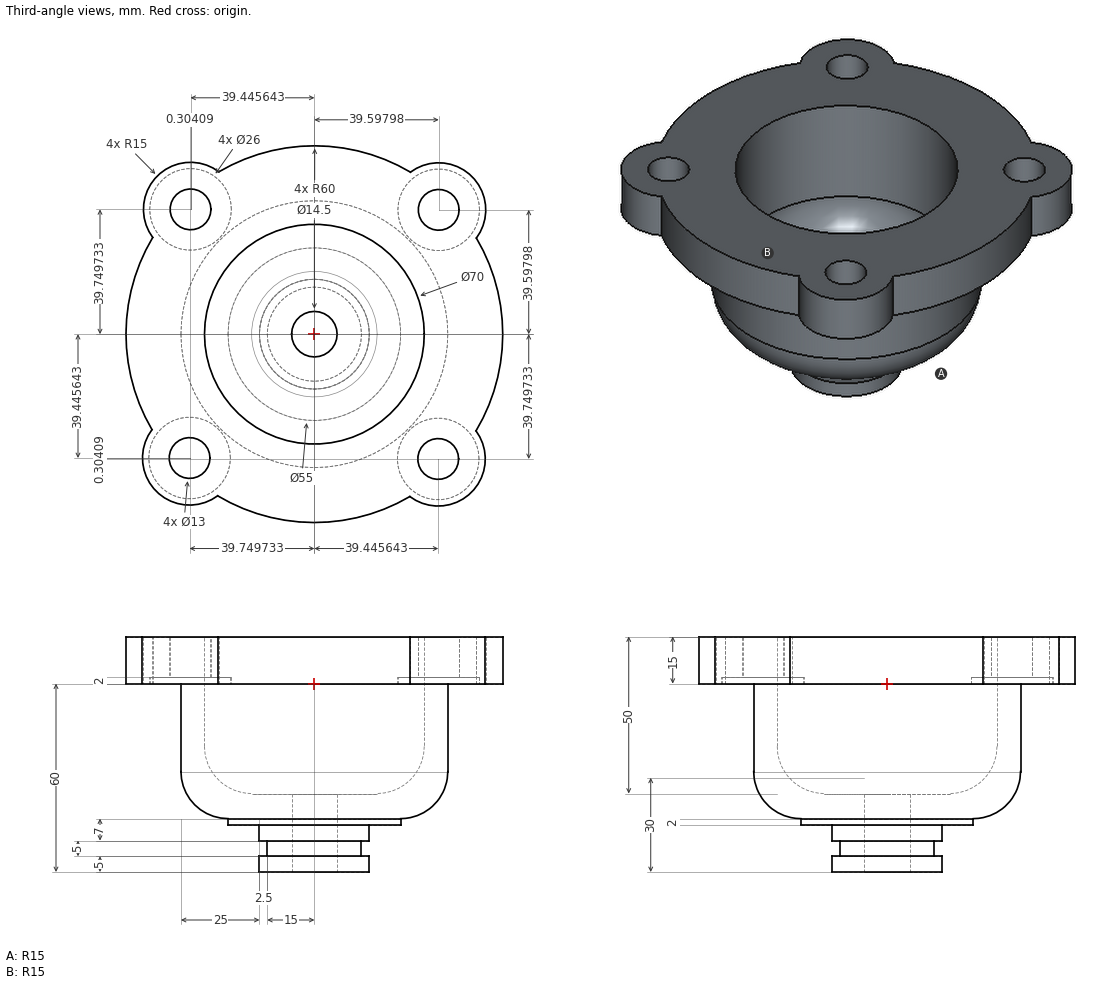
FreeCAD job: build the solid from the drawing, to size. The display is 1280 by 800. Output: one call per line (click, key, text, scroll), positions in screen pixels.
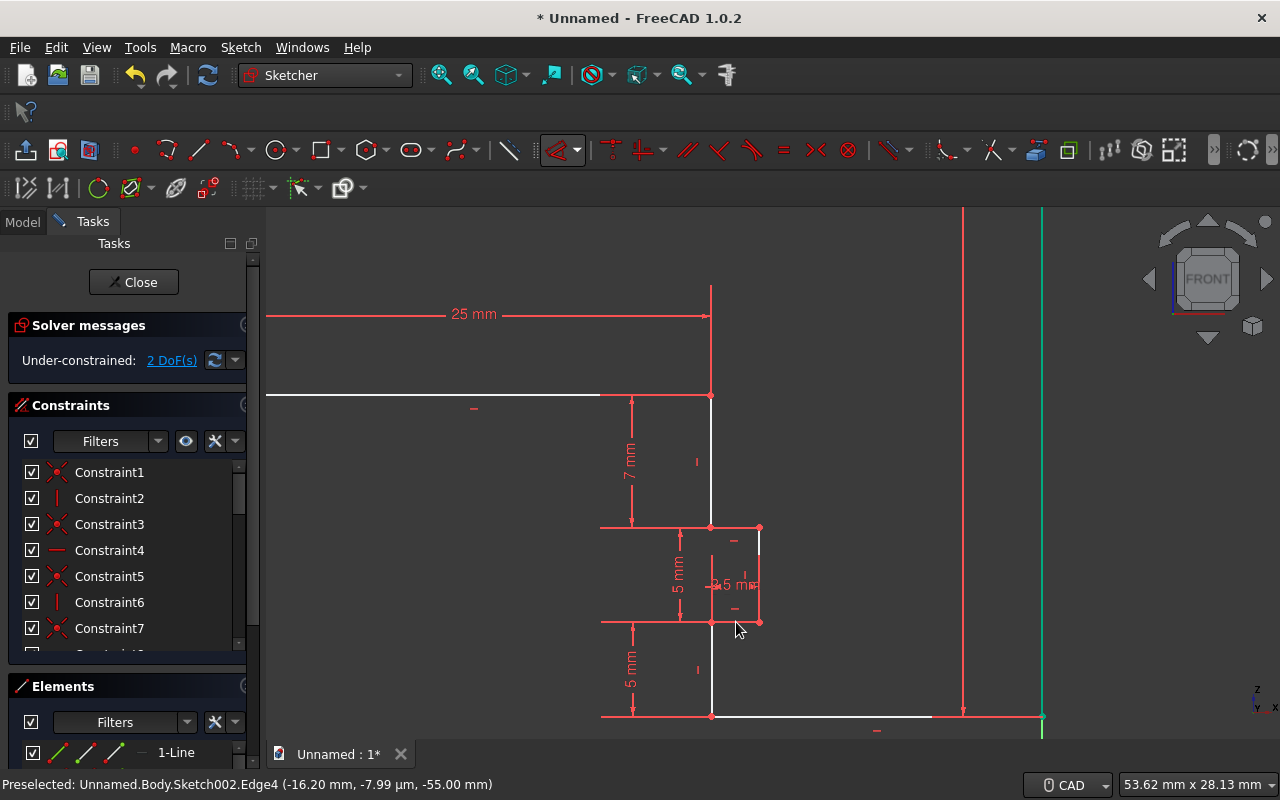
click(745, 528)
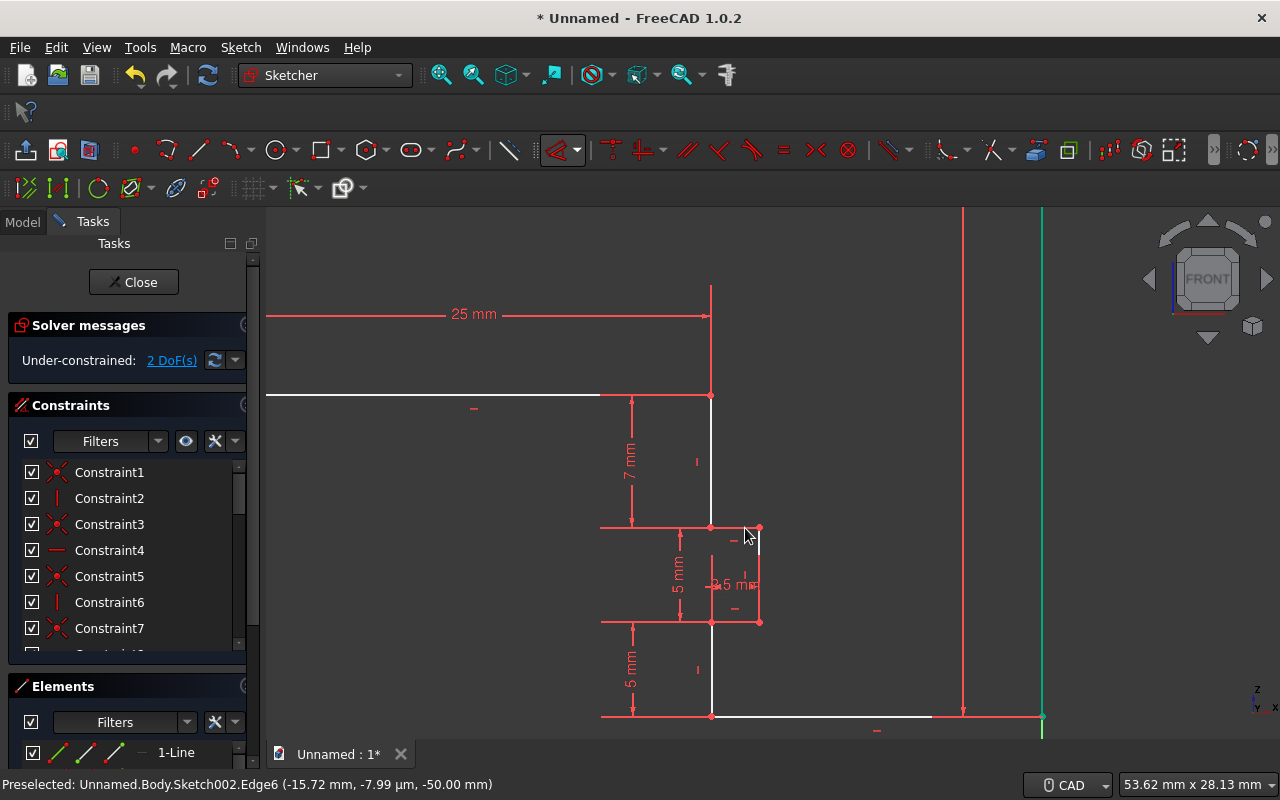
key(l)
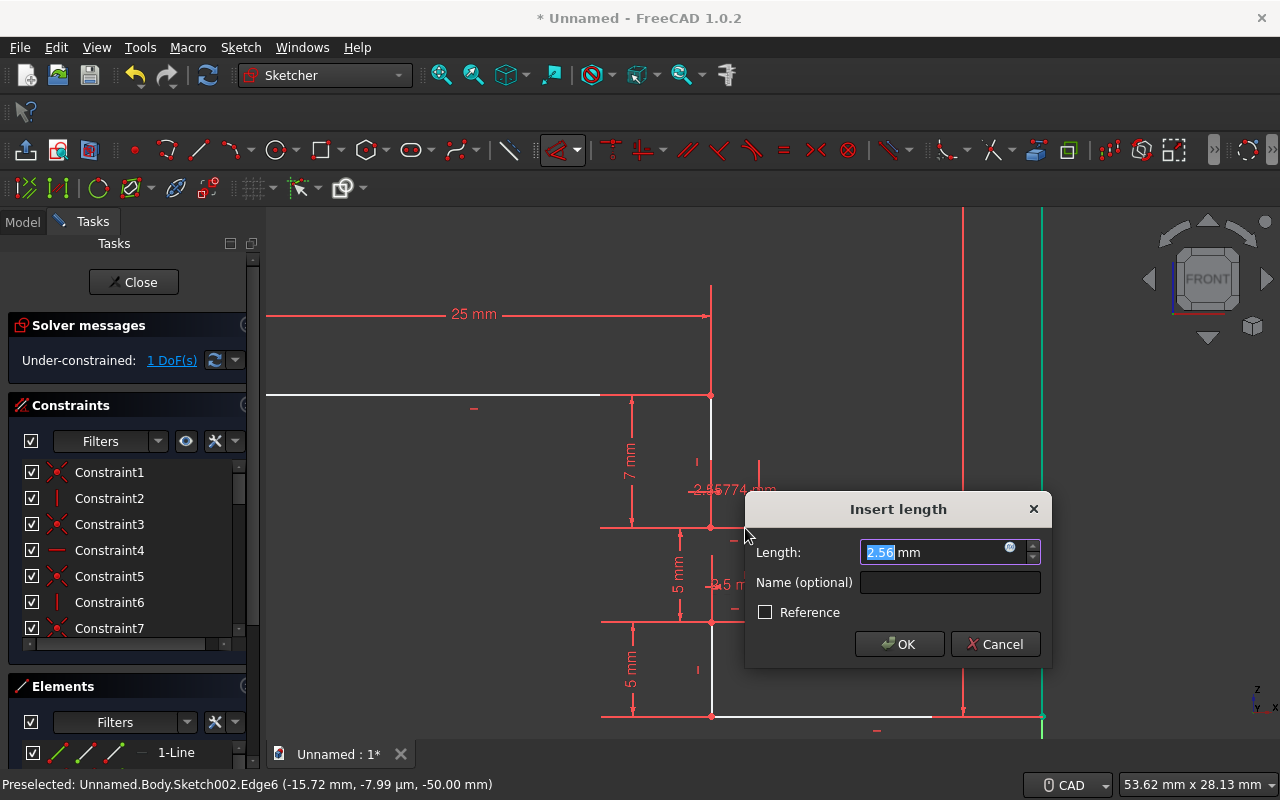
text(2.5)
key(Return)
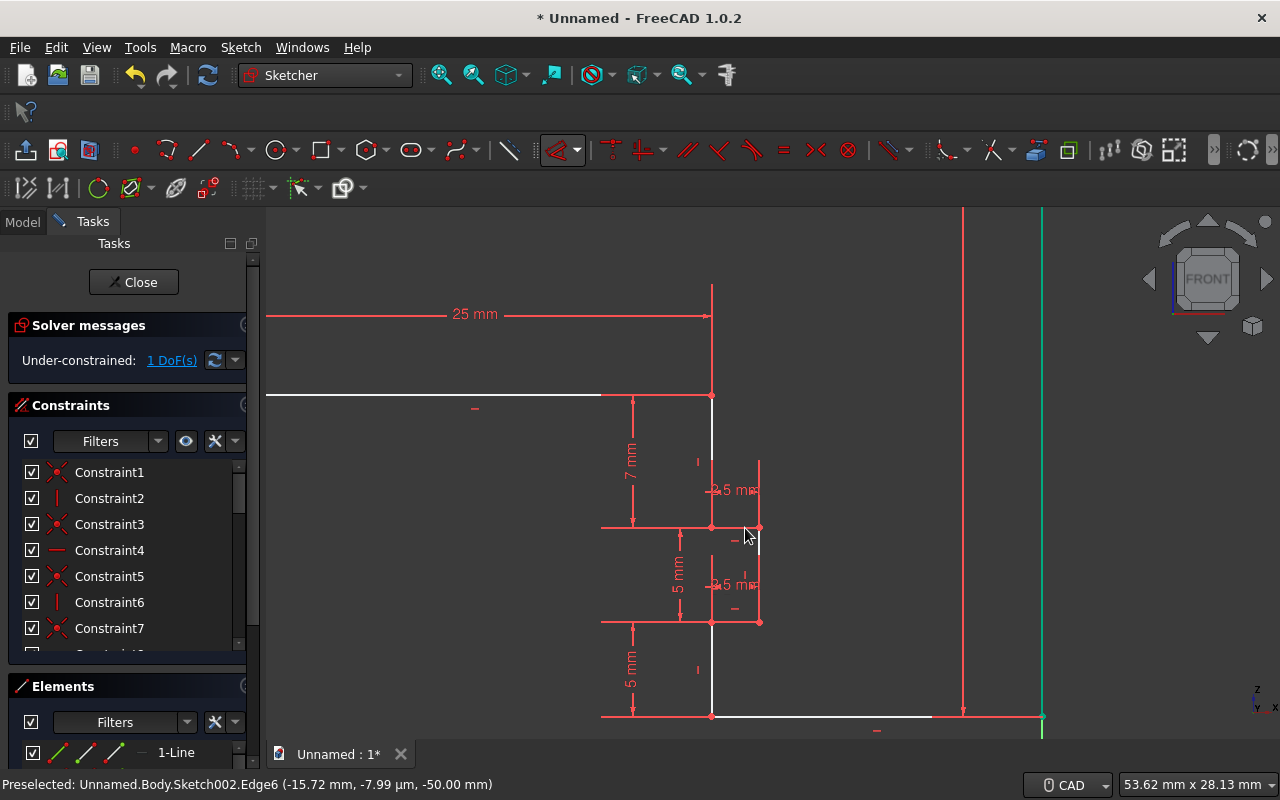
click(759, 622)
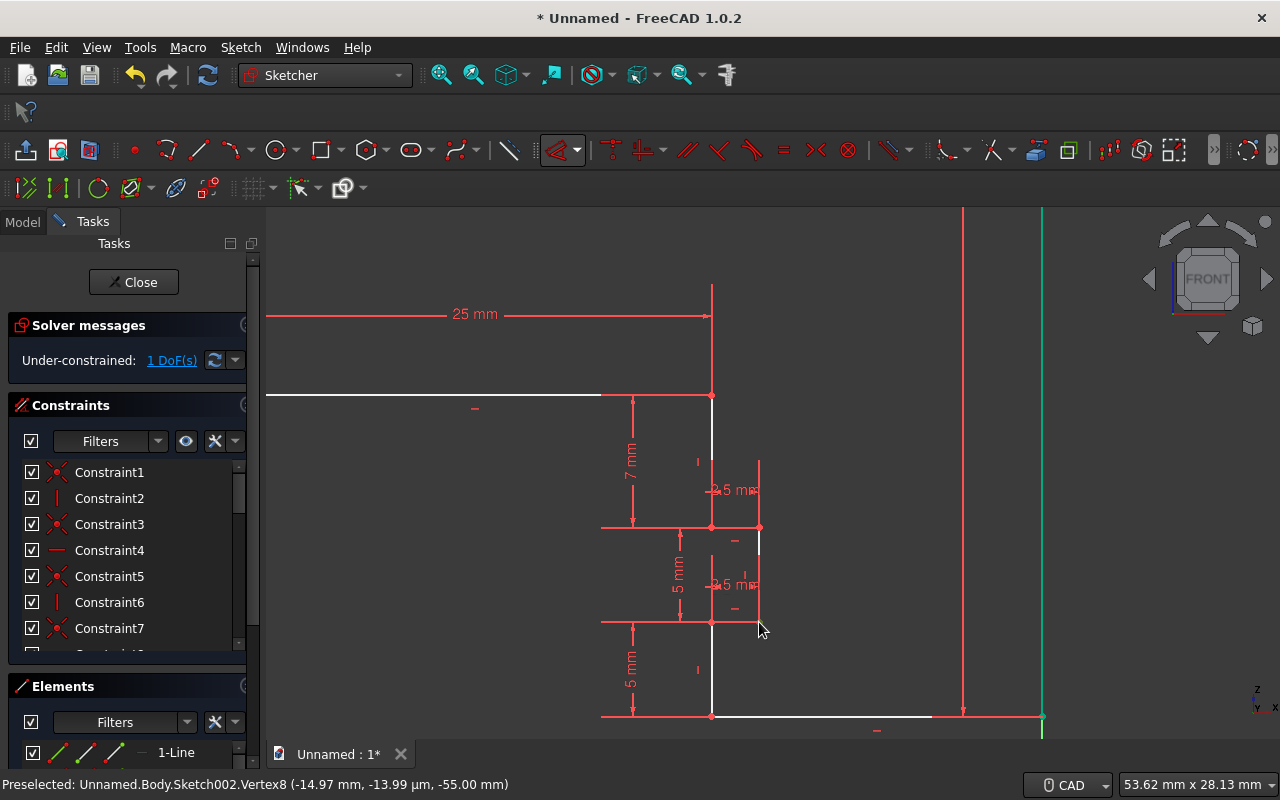
key(l)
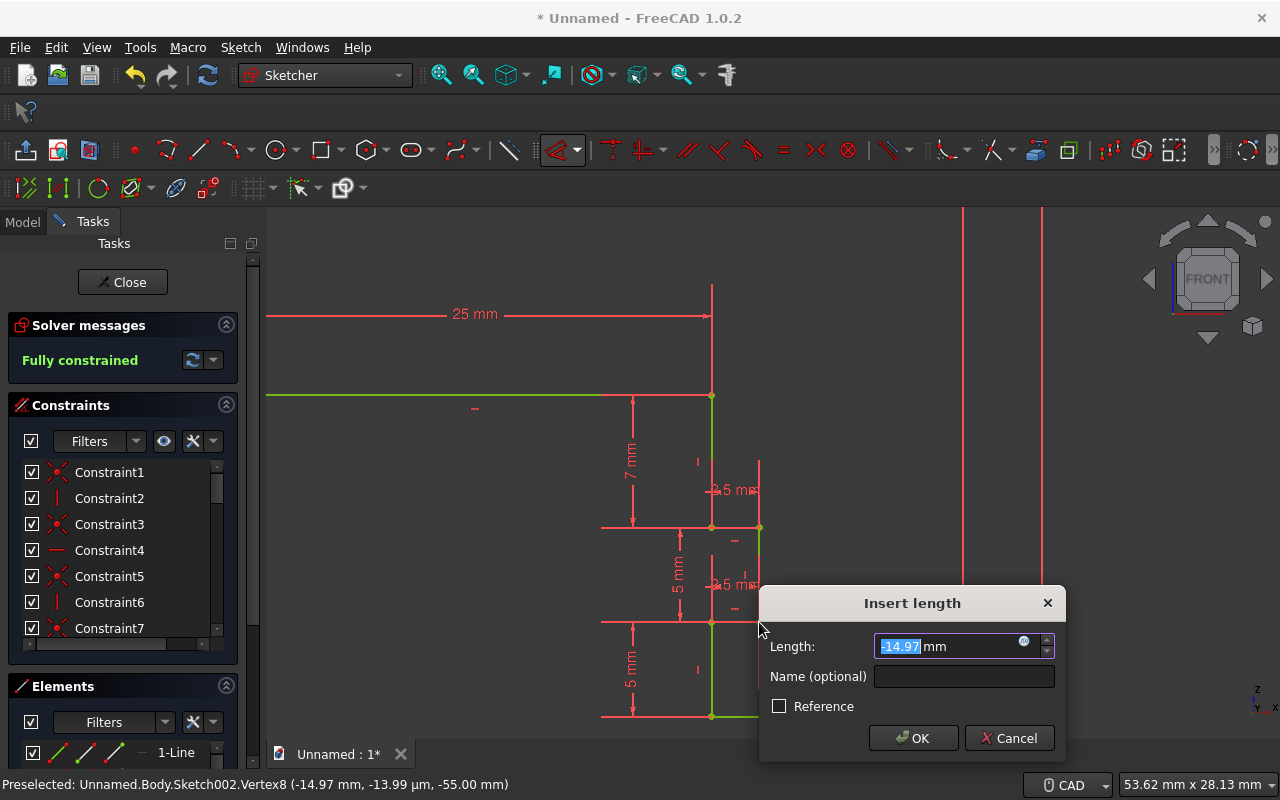
text(-15)
key(Return)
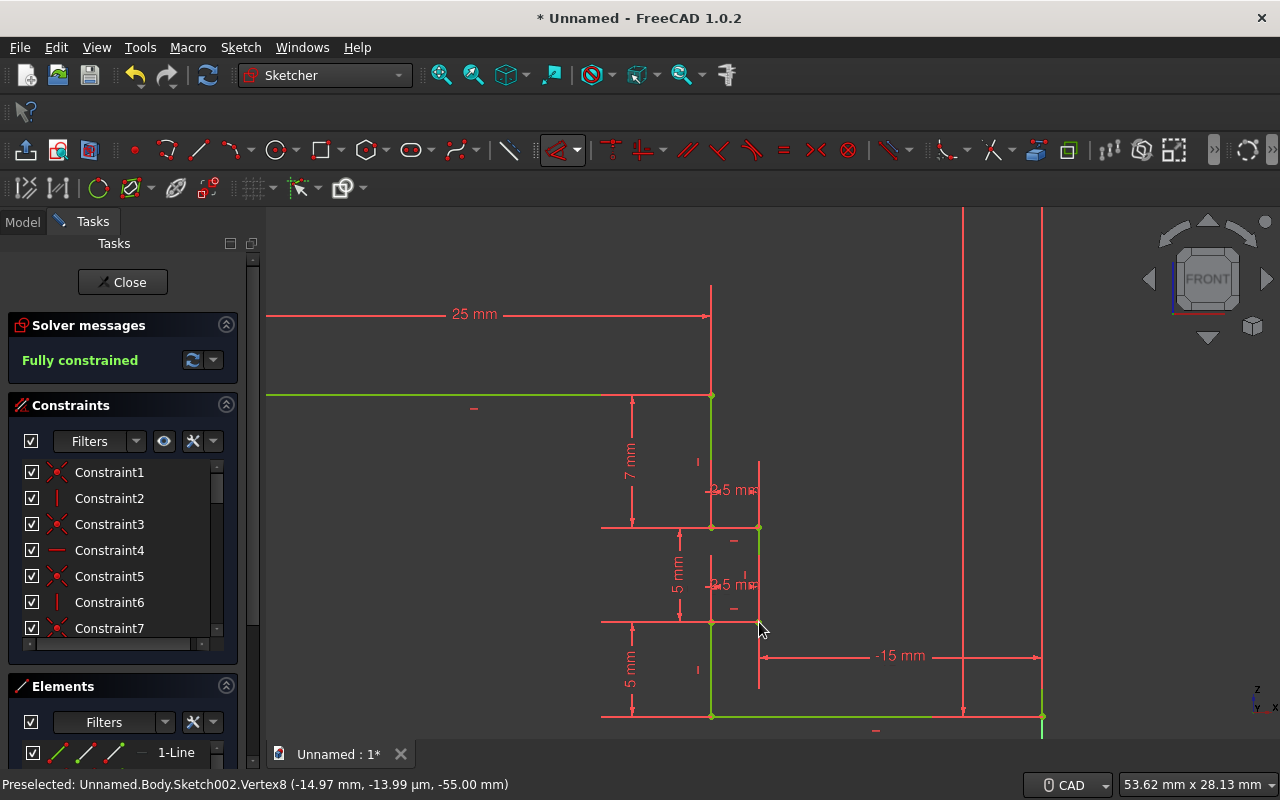
click(123, 282)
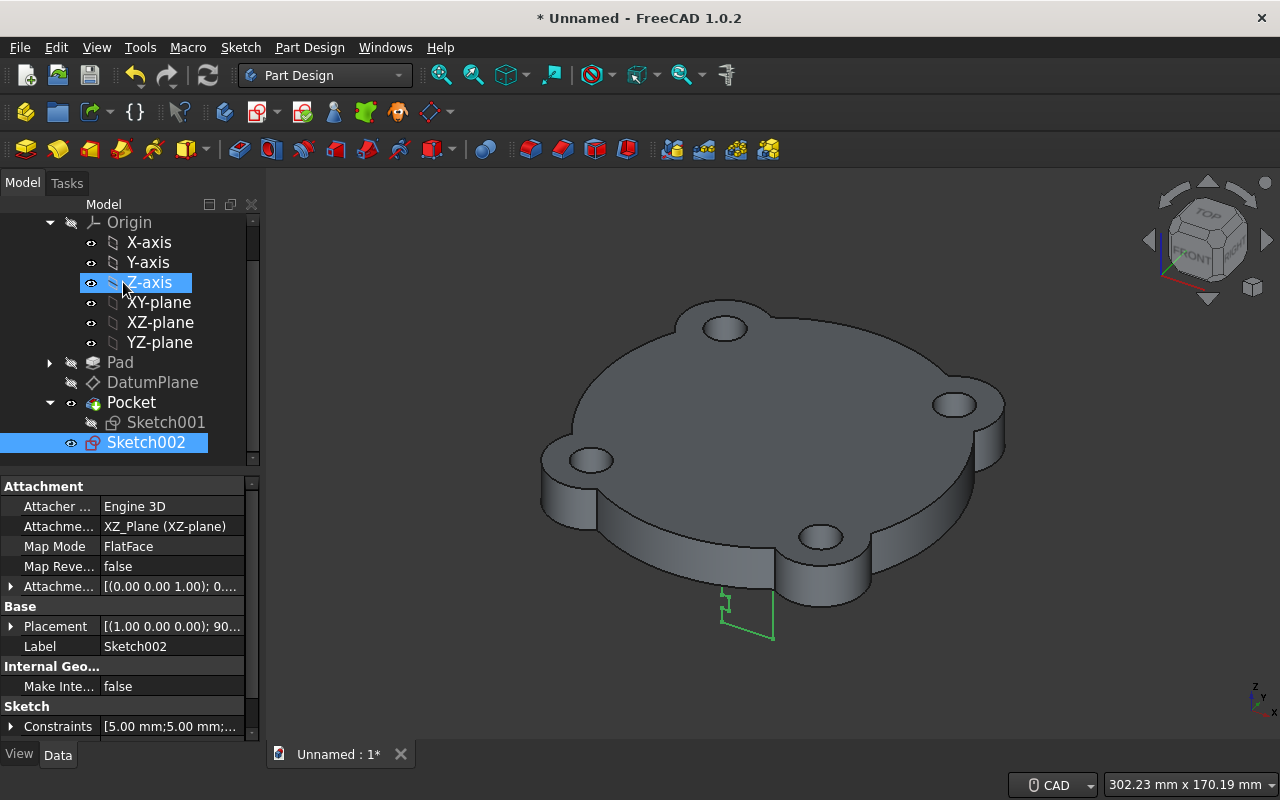
click(58, 150)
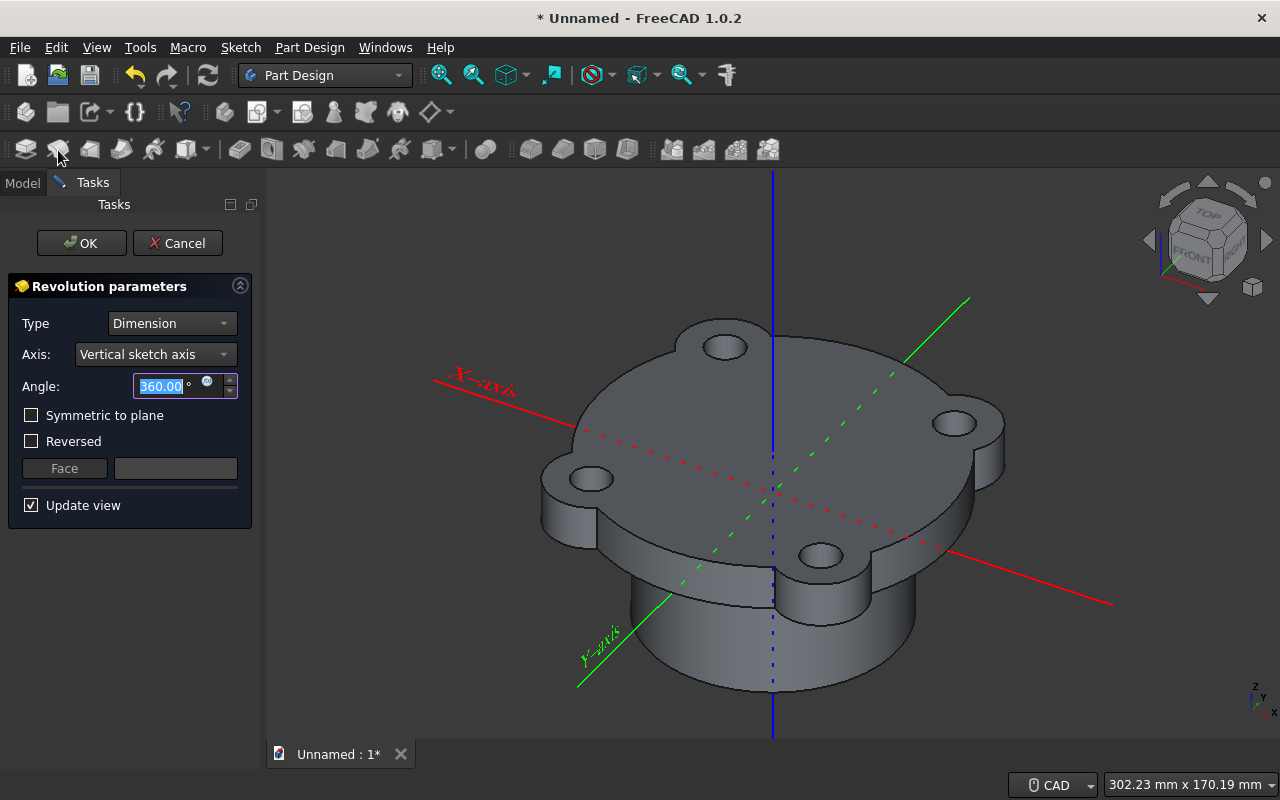
click(82, 243)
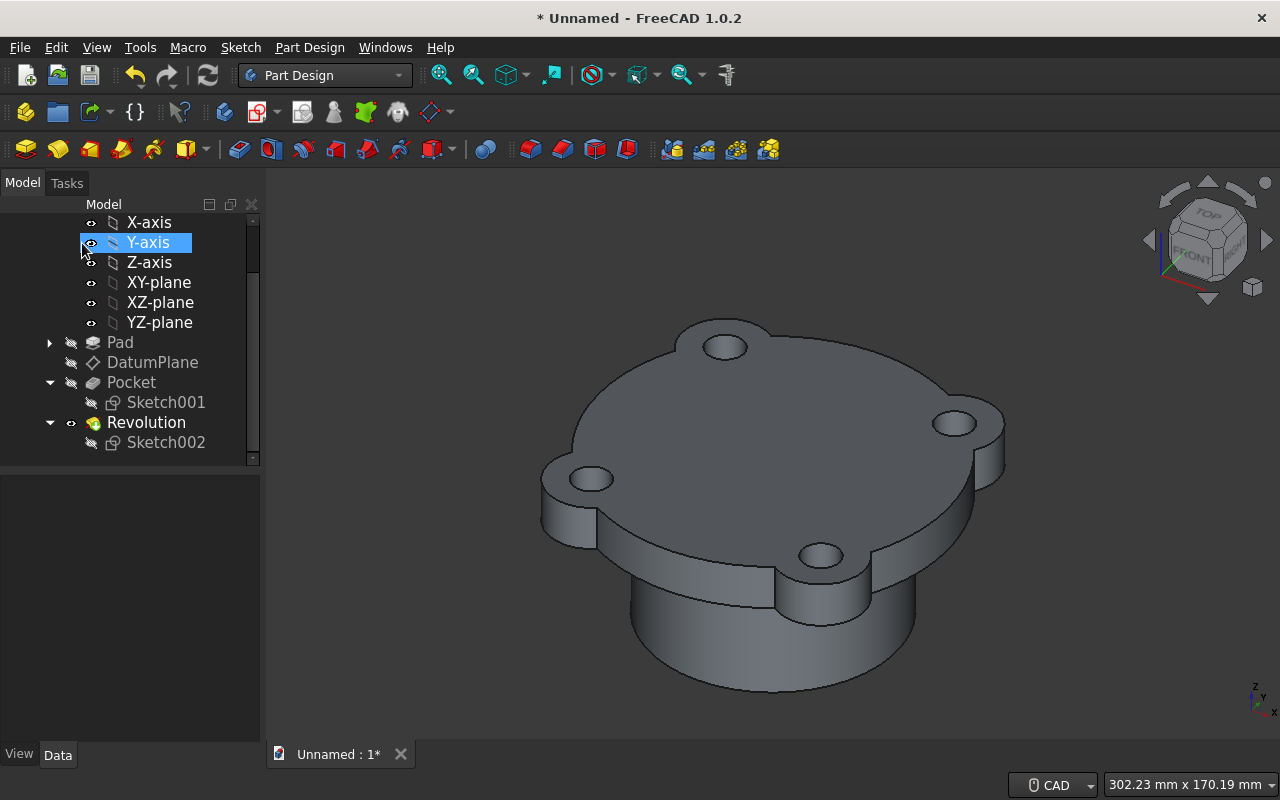
click(442, 76)